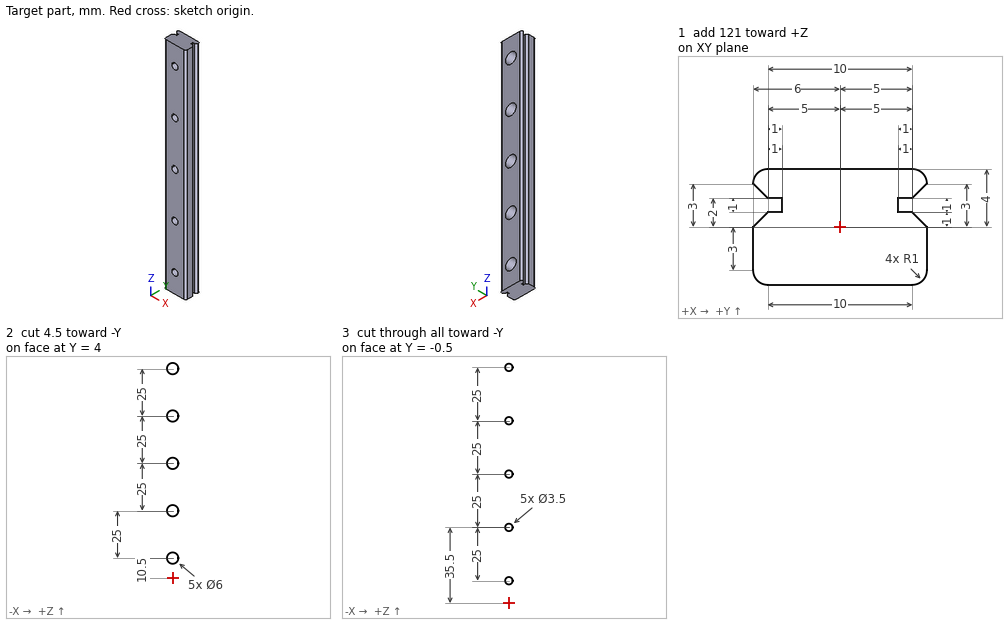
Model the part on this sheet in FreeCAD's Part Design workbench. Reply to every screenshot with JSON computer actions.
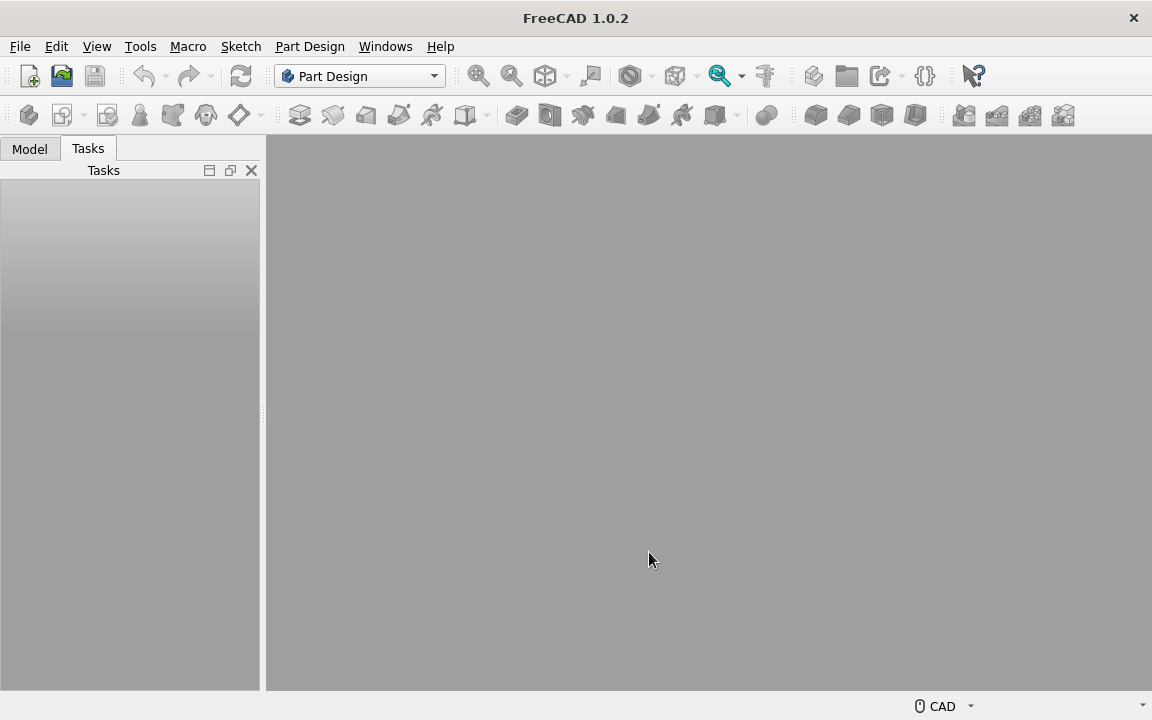
{"action": "left_click", "coordinate": [29, 76]}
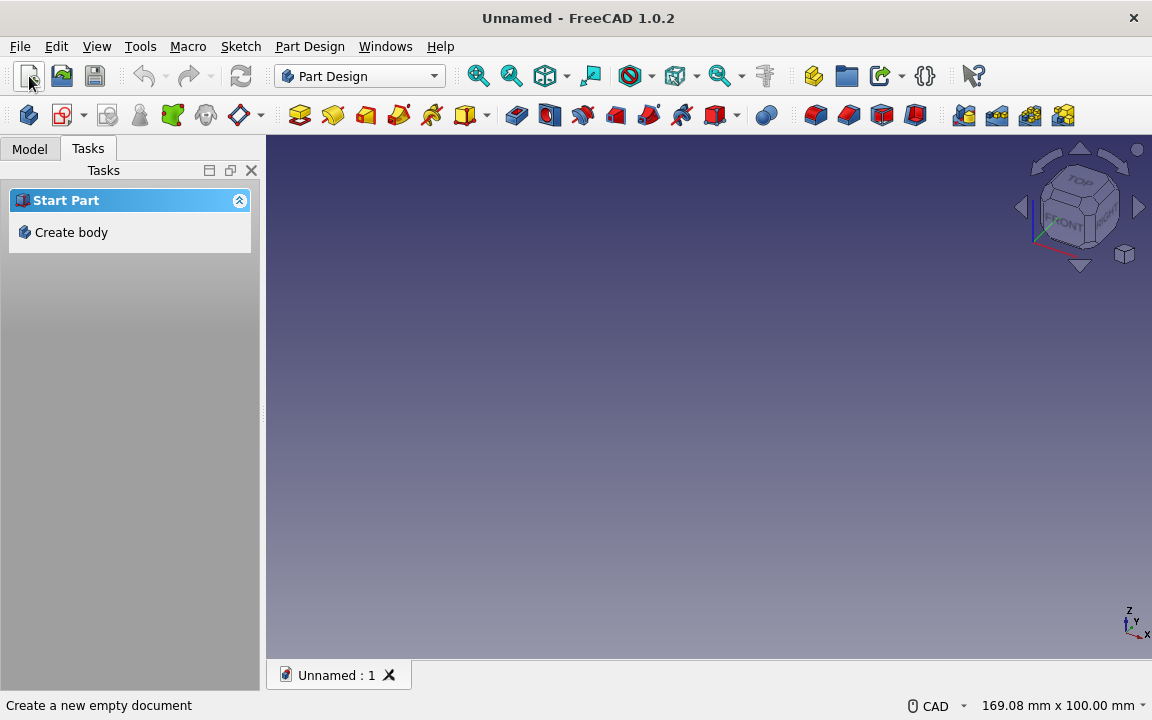
{"action": "left_click", "coordinate": [62, 116]}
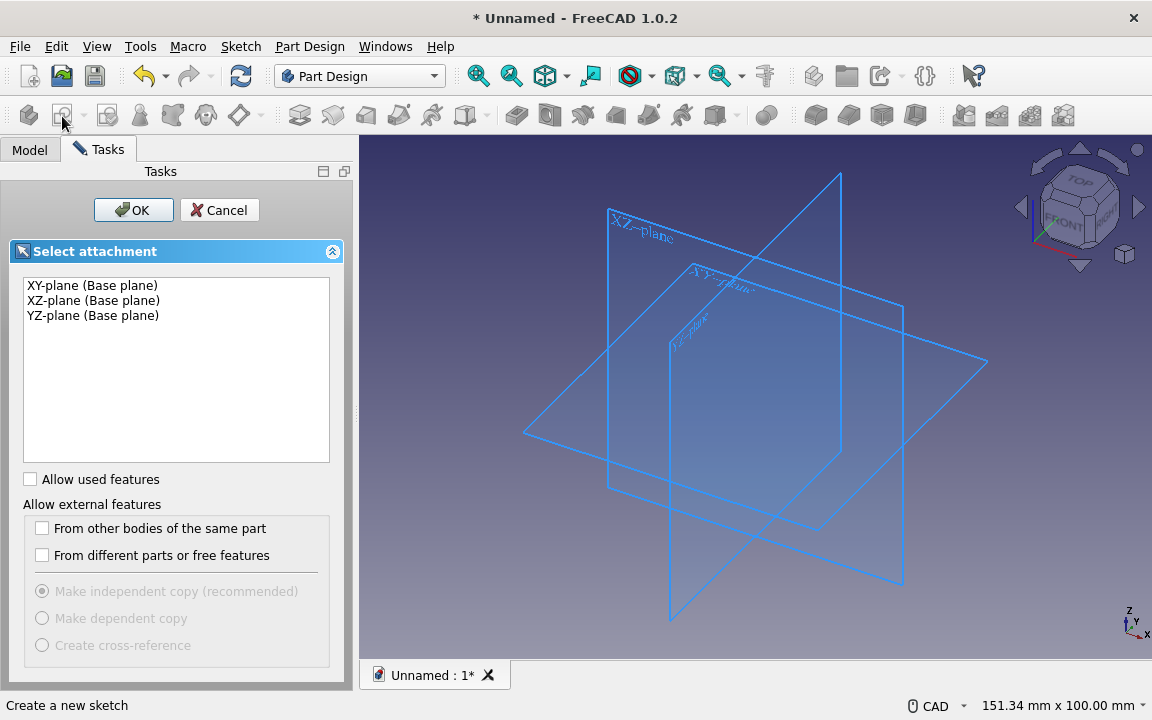
{"action": "left_click", "coordinate": [84, 286]}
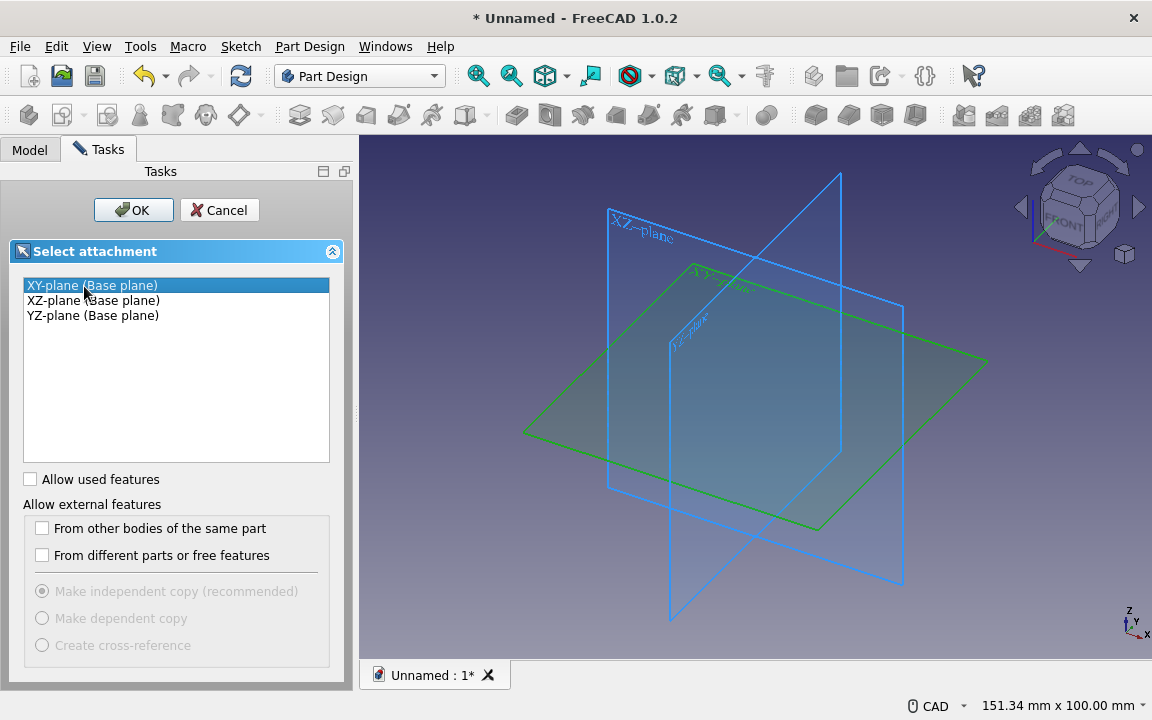
{"action": "left_click", "coordinate": [134, 210]}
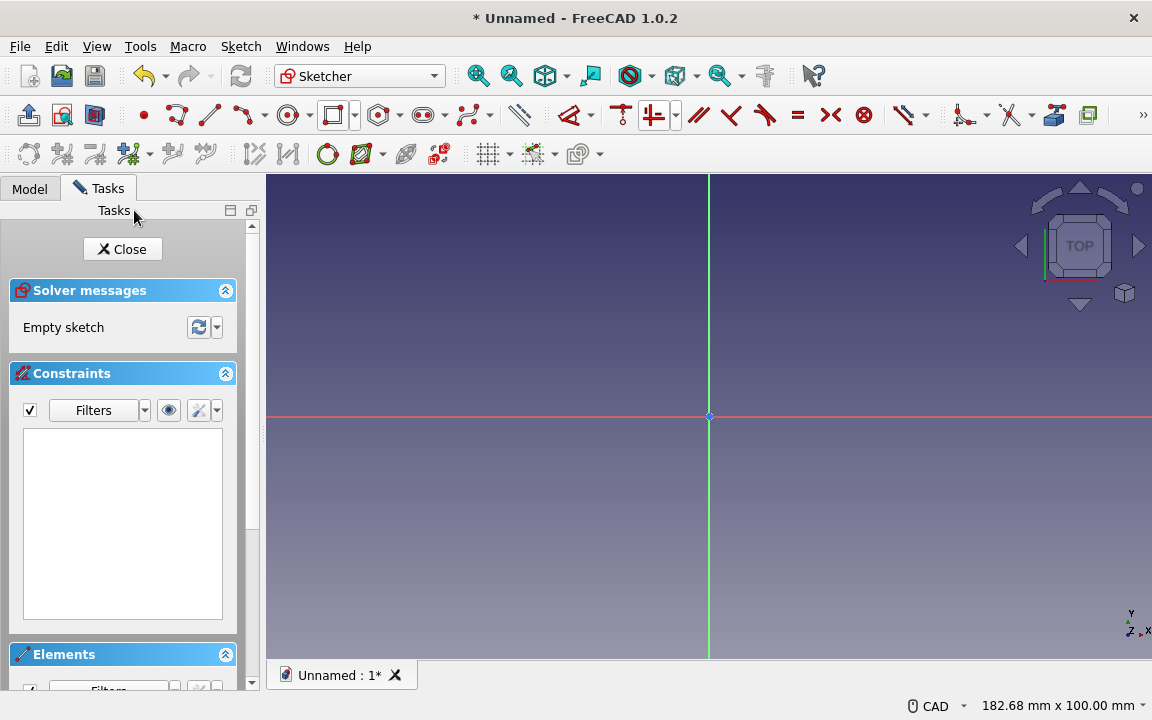
{"action": "scroll", "coordinate": [720, 416], "scroll_direction": "up", "scroll_amount": 10}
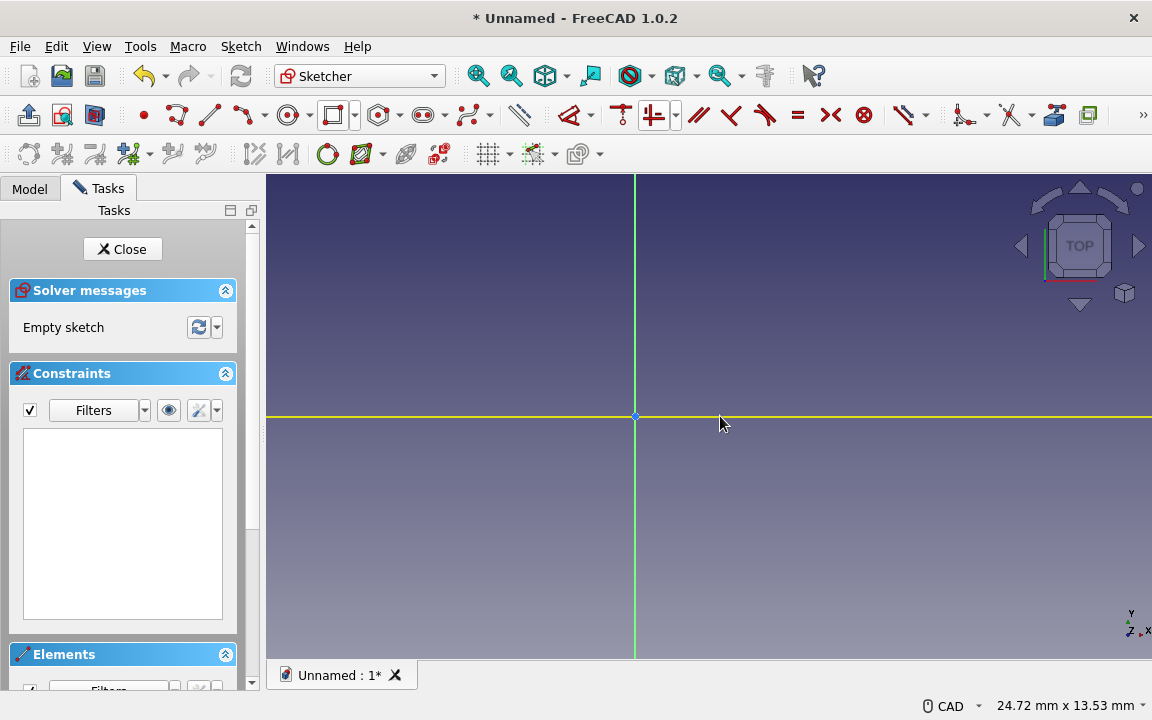
{"action": "left_click", "coordinate": [210, 116]}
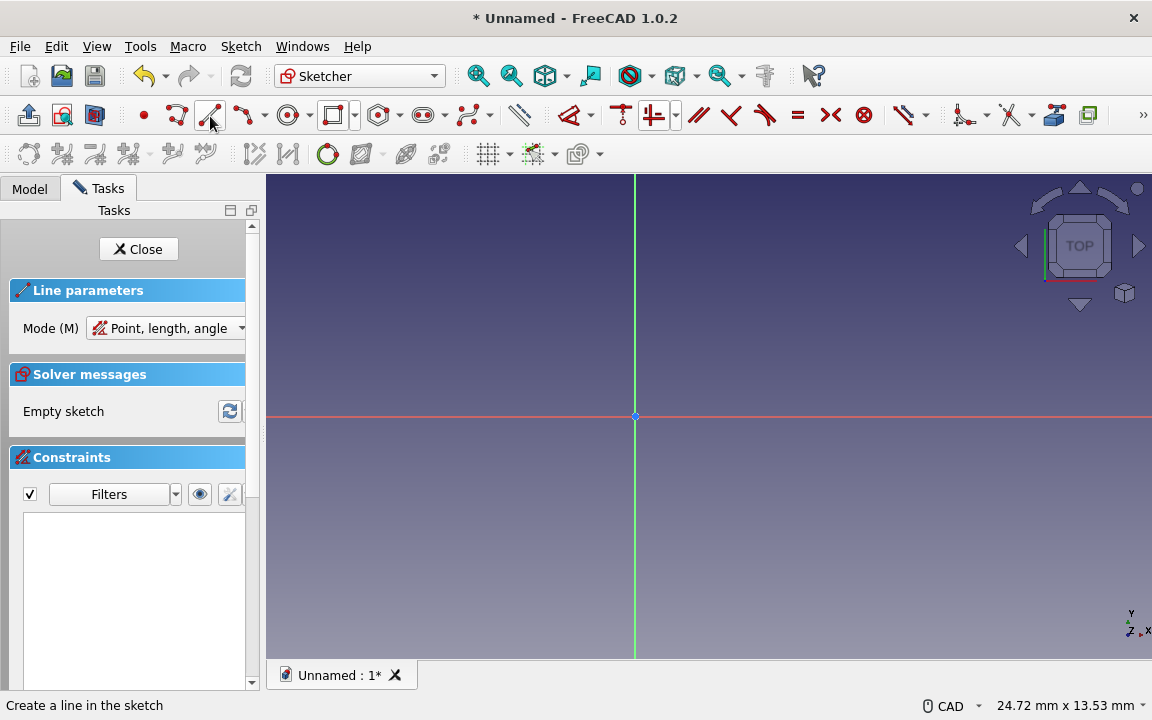
{"action": "left_click", "coordinate": [815, 273]}
{"action": "left_click", "coordinate": [456, 273]}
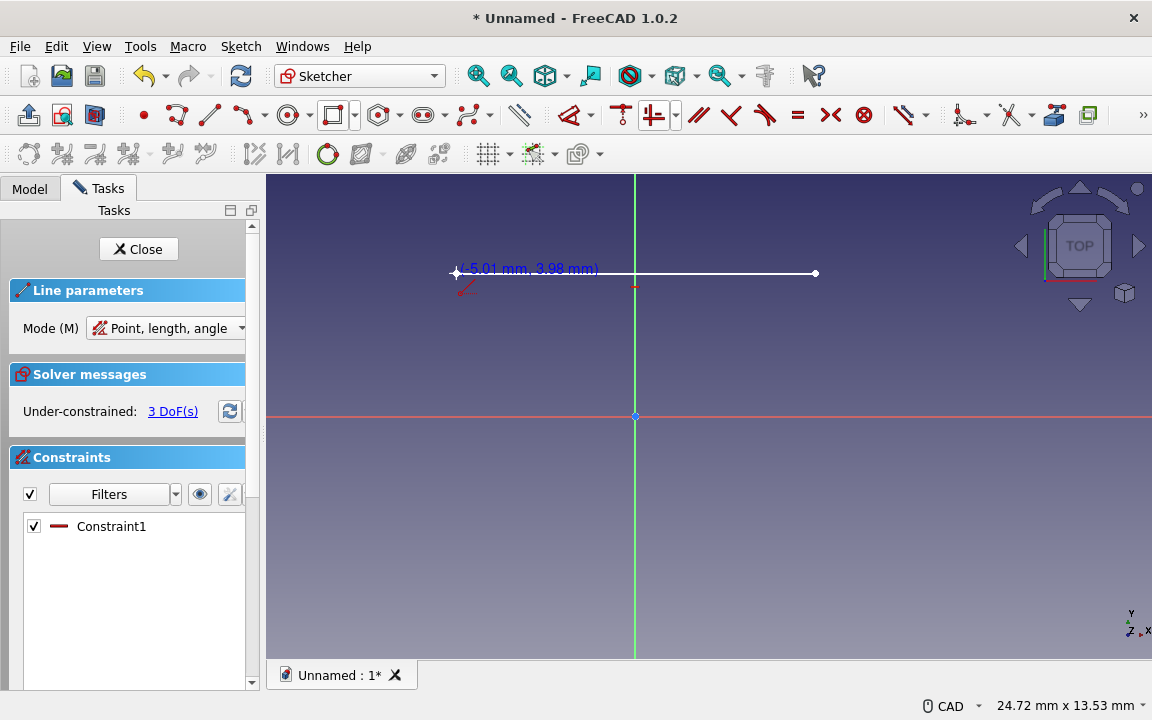
{"action": "left_click", "coordinate": [177, 116]}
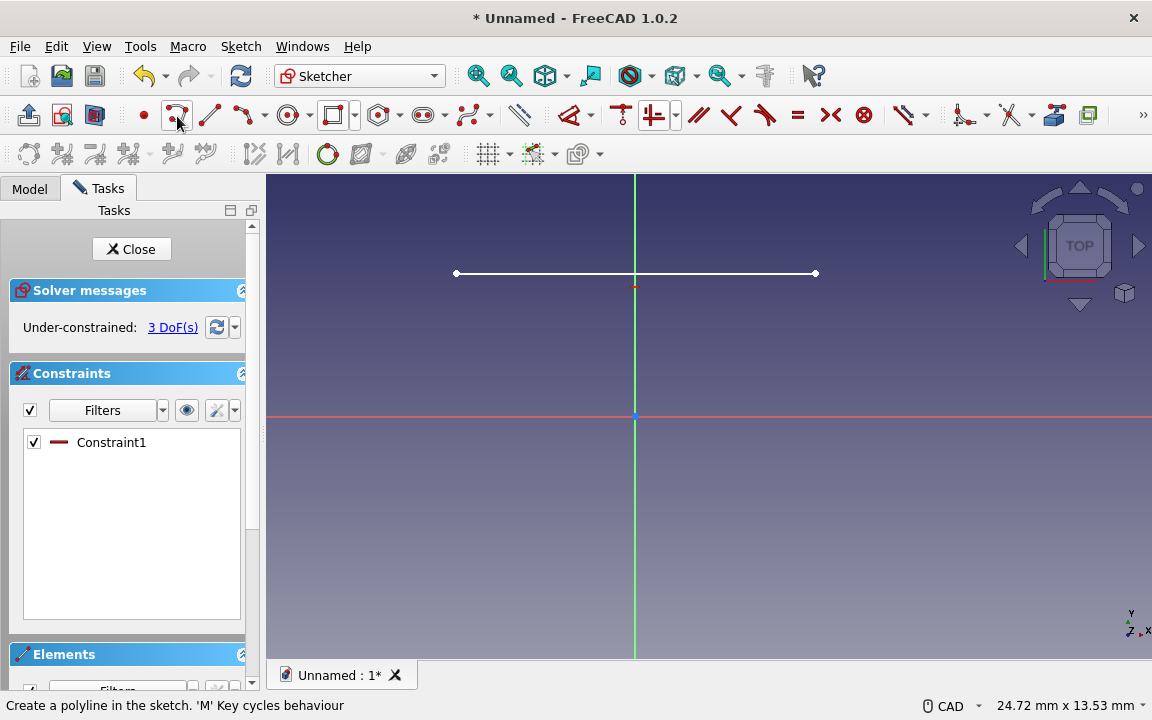
{"action": "left_click", "coordinate": [420, 309]}
{"action": "left_click", "coordinate": [456, 345]}
{"action": "left_click", "coordinate": [492, 345]}
{"action": "left_click", "coordinate": [492, 381]}
{"action": "left_click", "coordinate": [456, 381]}
{"action": "left_click", "coordinate": [420, 416]}
{"action": "left_click", "coordinate": [420, 524]}
{"action": "right_click", "coordinate": [420, 524]}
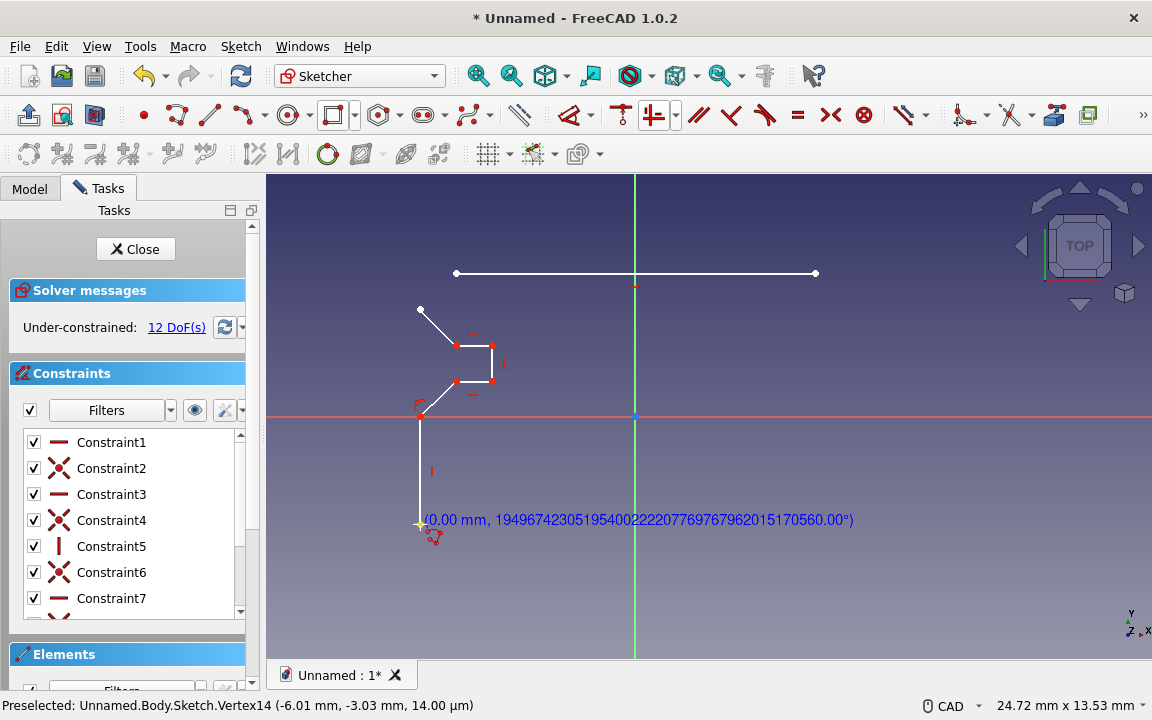
{"action": "left_click", "coordinate": [210, 116]}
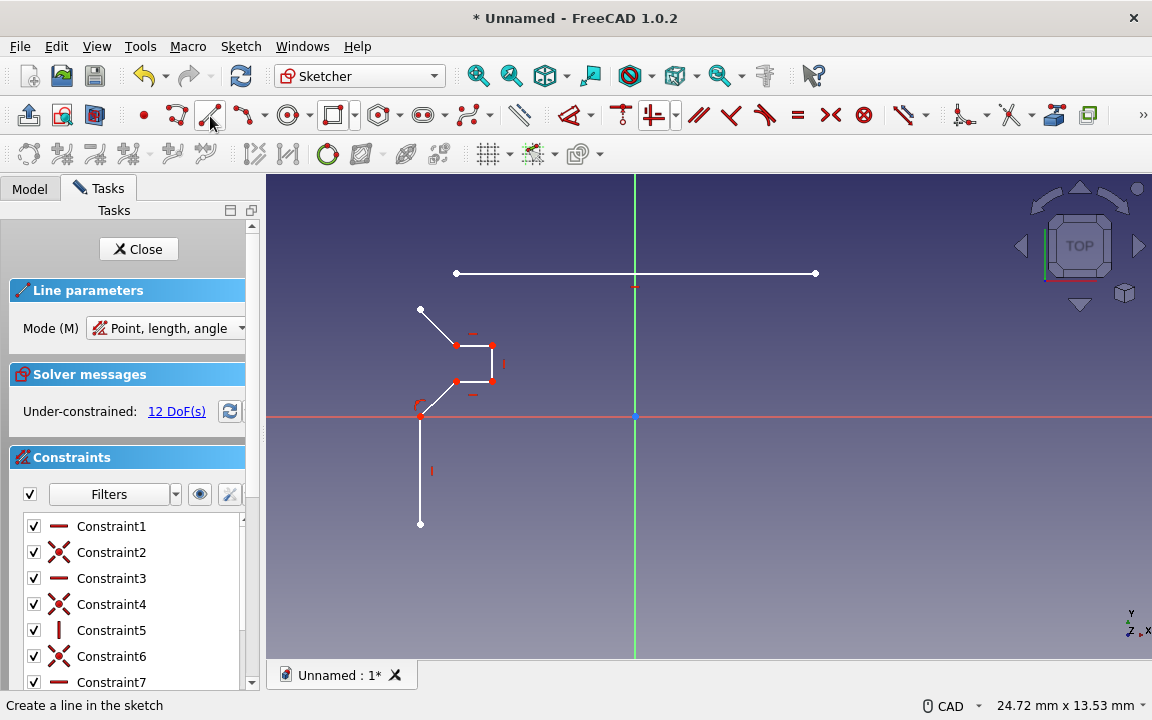
{"action": "left_click", "coordinate": [456, 560]}
{"action": "left_click", "coordinate": [815, 560]}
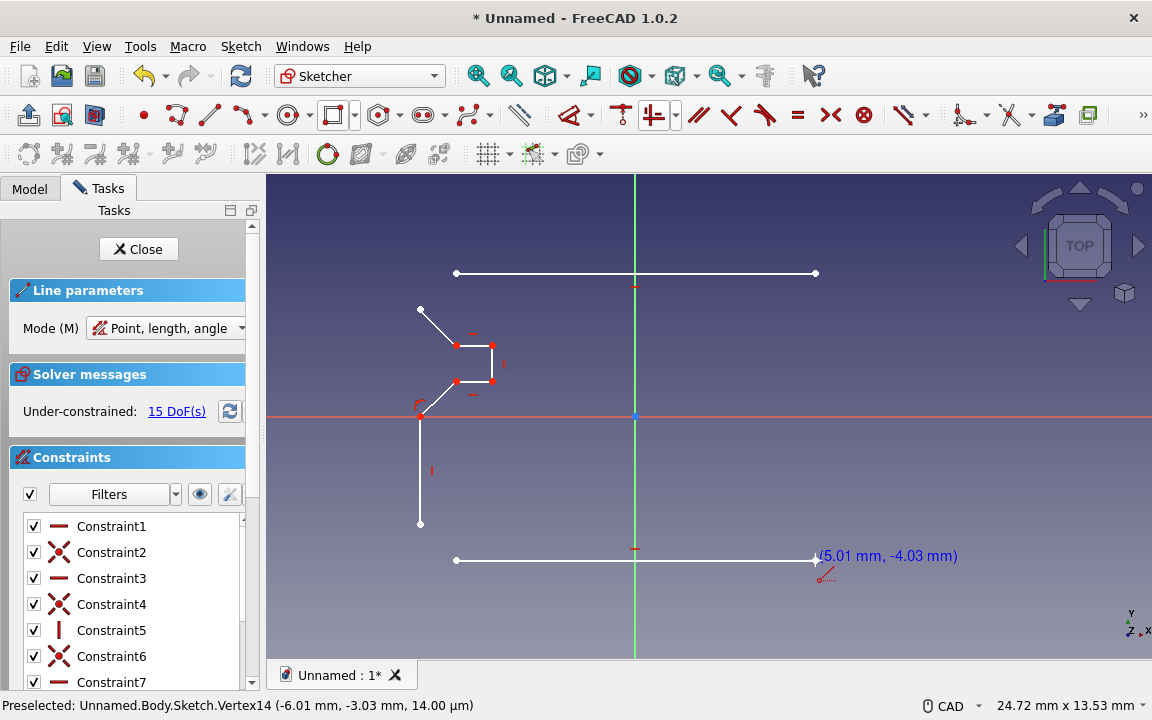
{"action": "left_click", "coordinate": [177, 116]}